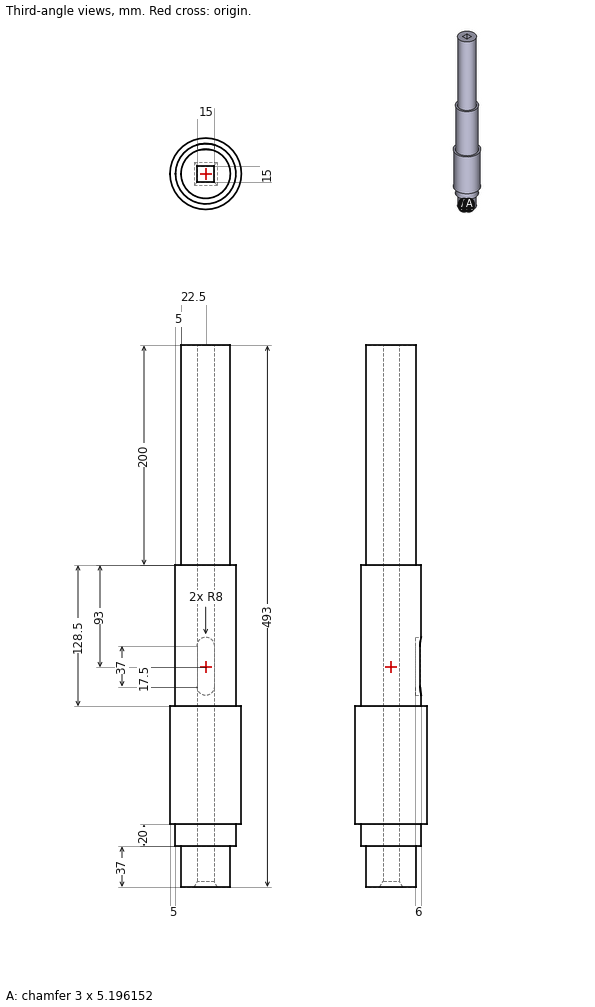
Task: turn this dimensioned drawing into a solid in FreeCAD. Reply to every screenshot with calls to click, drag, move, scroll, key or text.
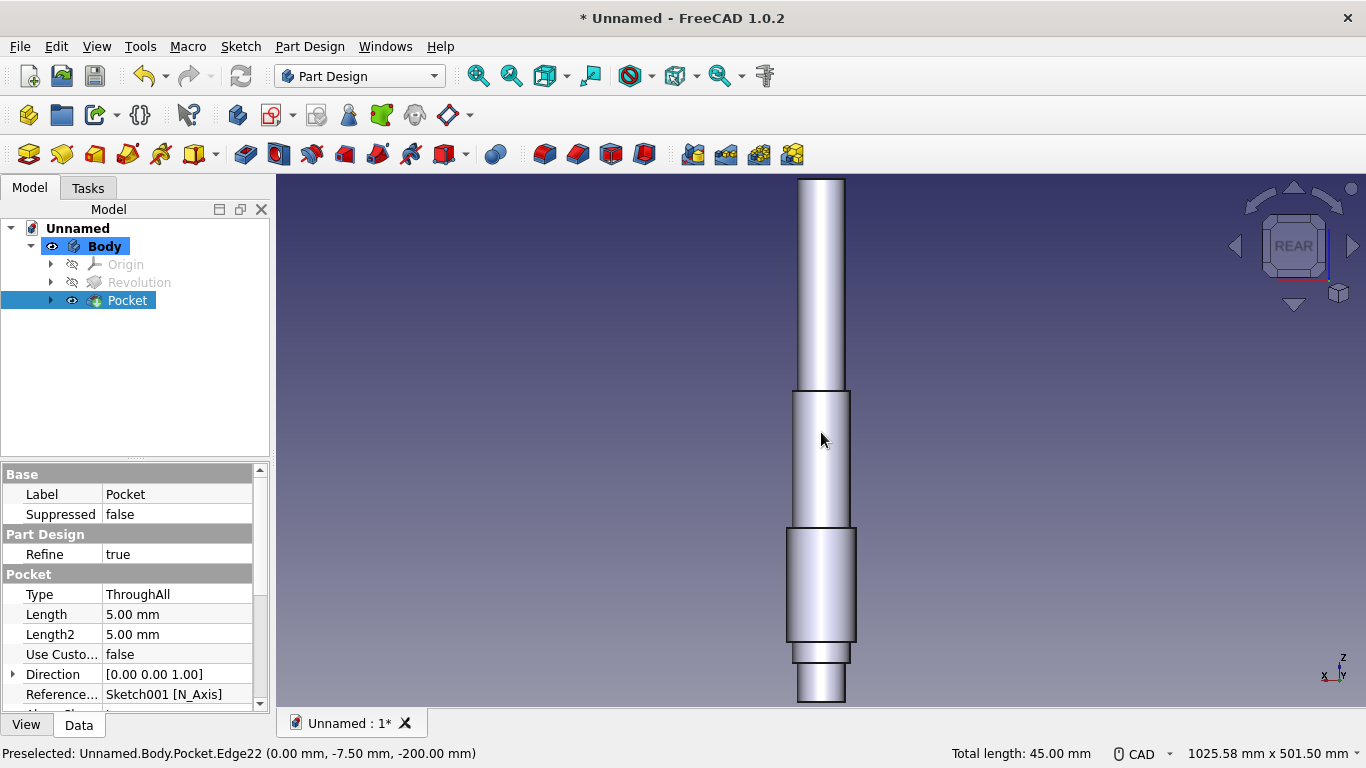
key(6)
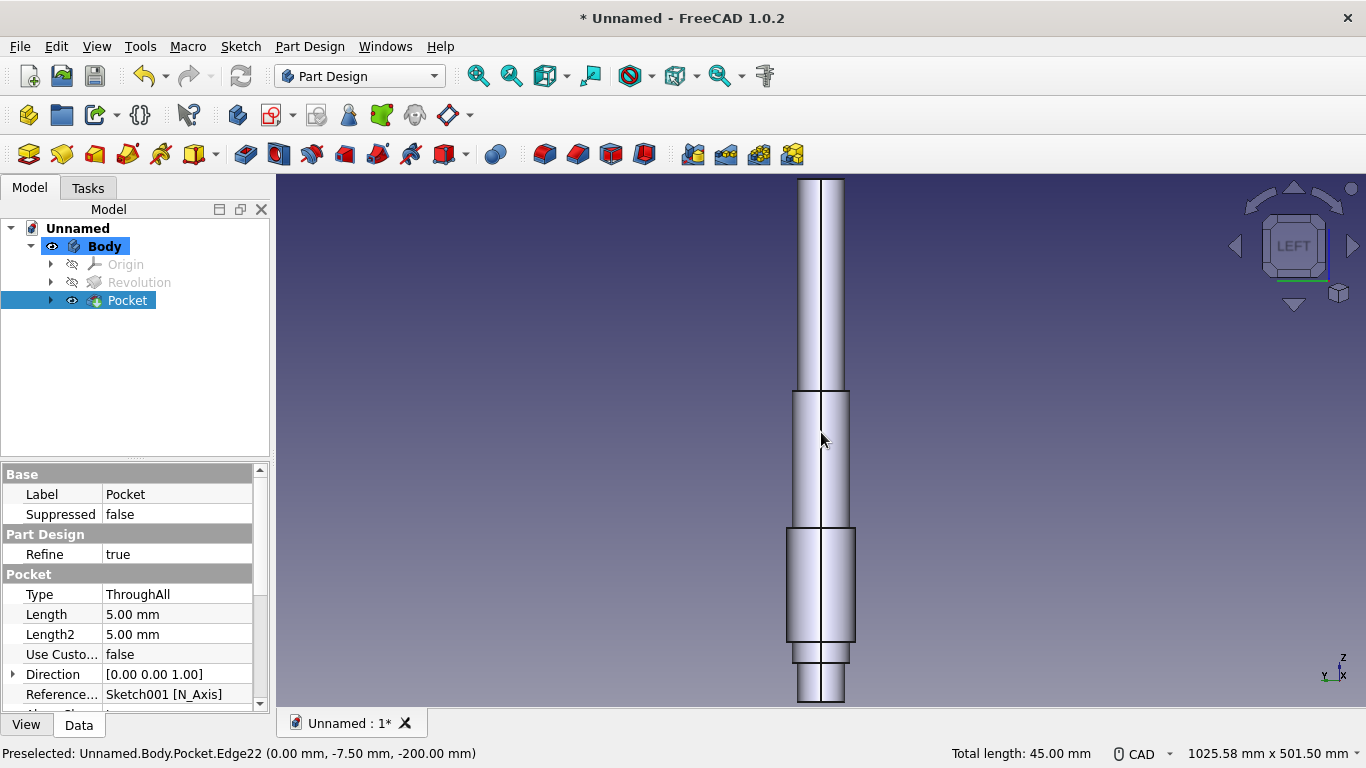
key(v)
key(3)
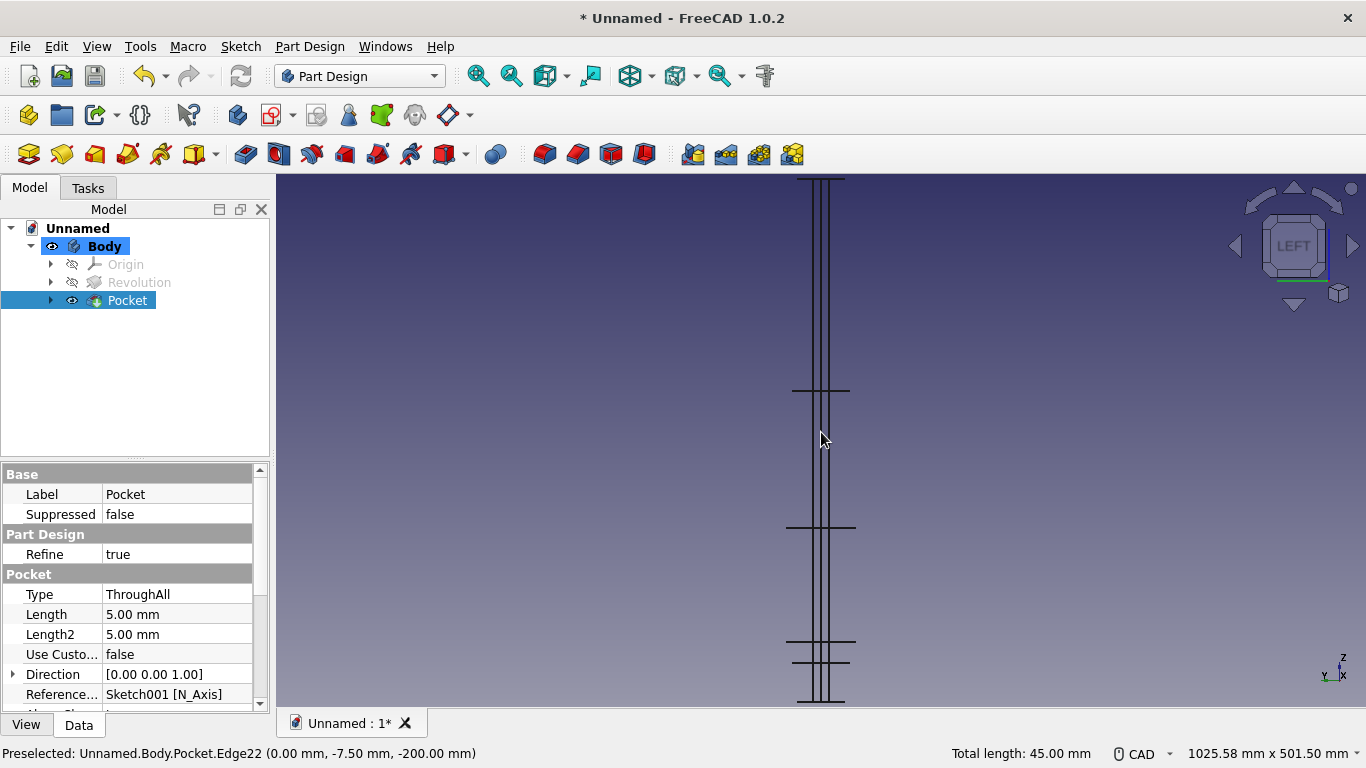
key(0)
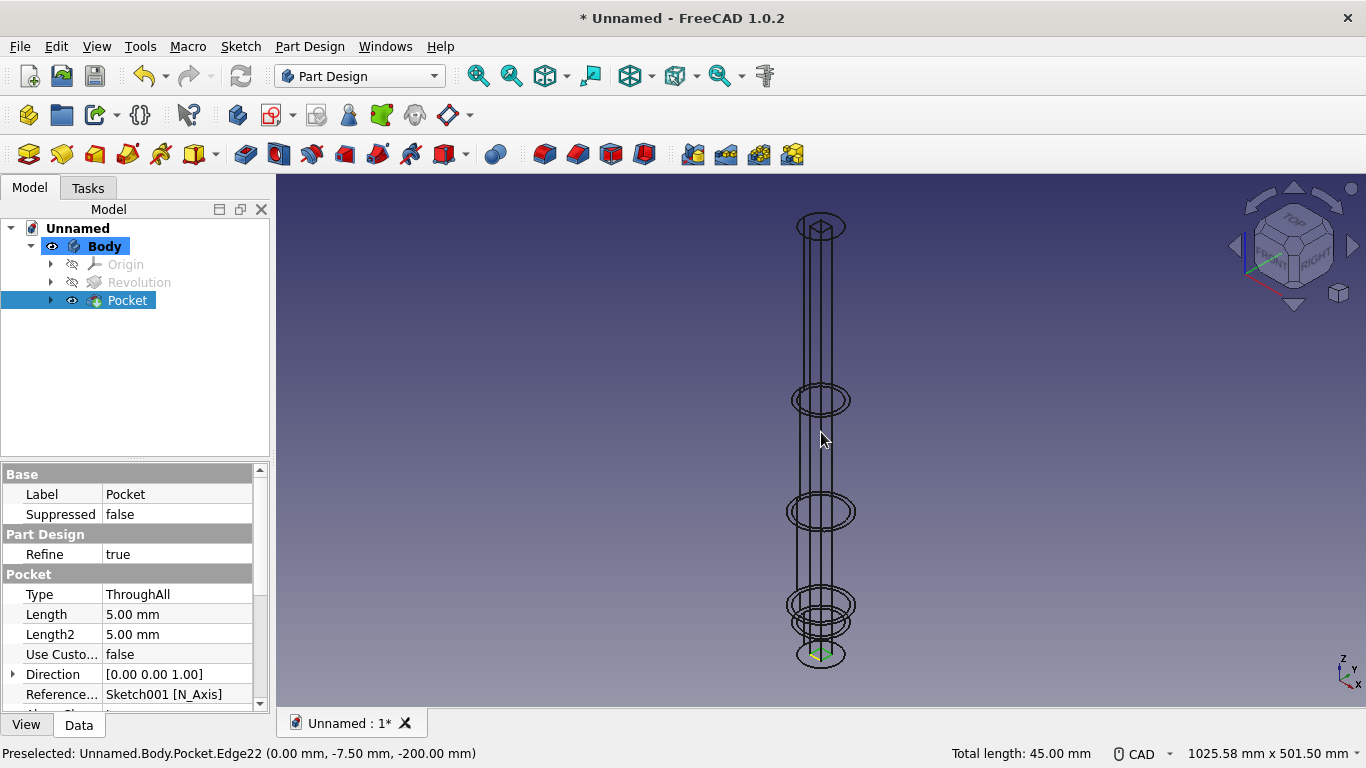
click(815, 657, ctrl)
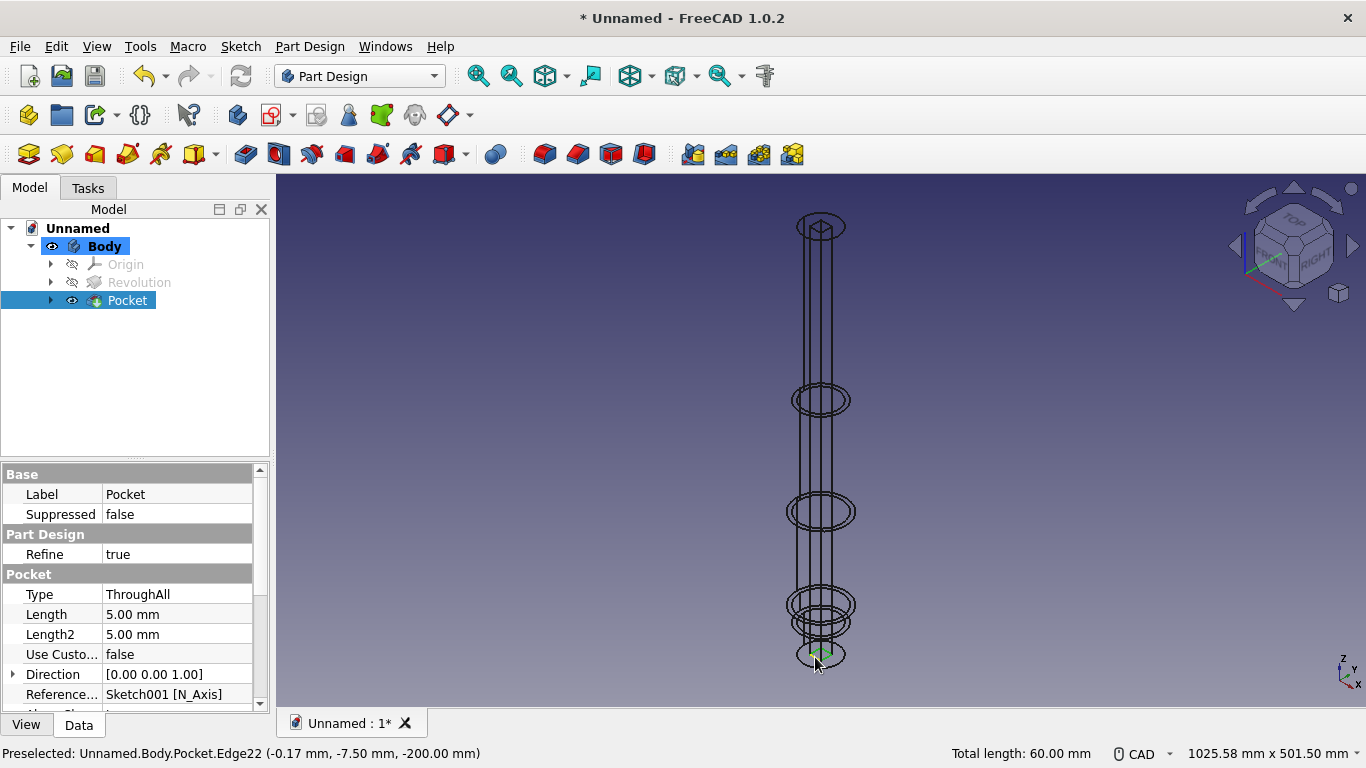
key(v)
key(1)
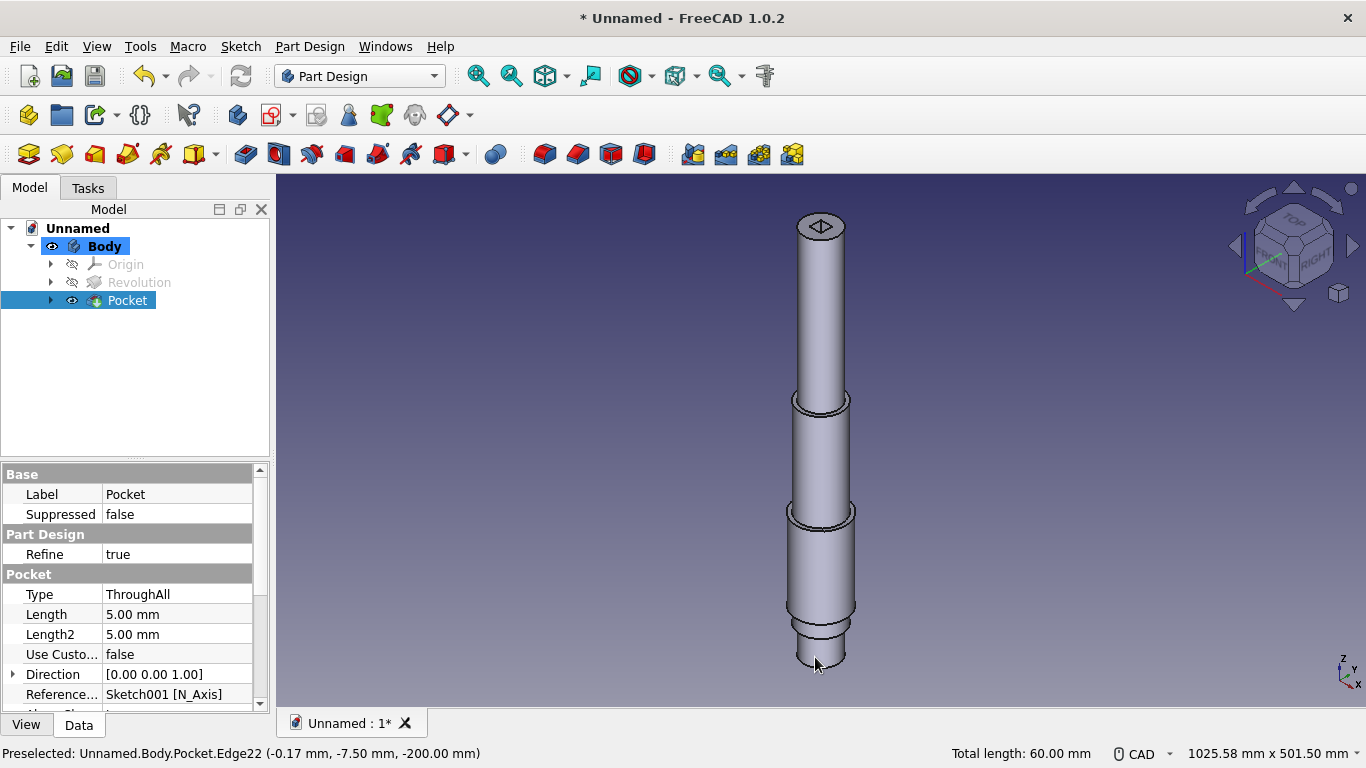
click(578, 154)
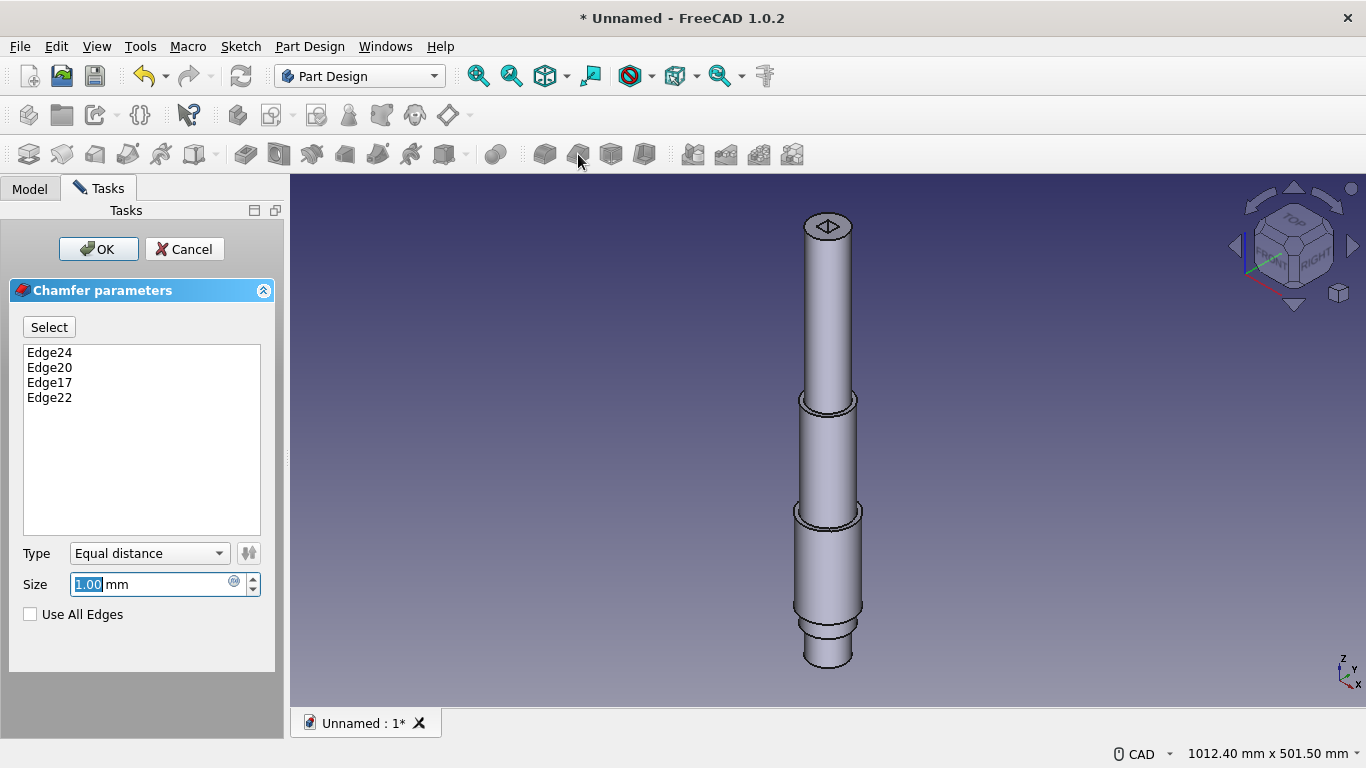
text(3)
key(Tab)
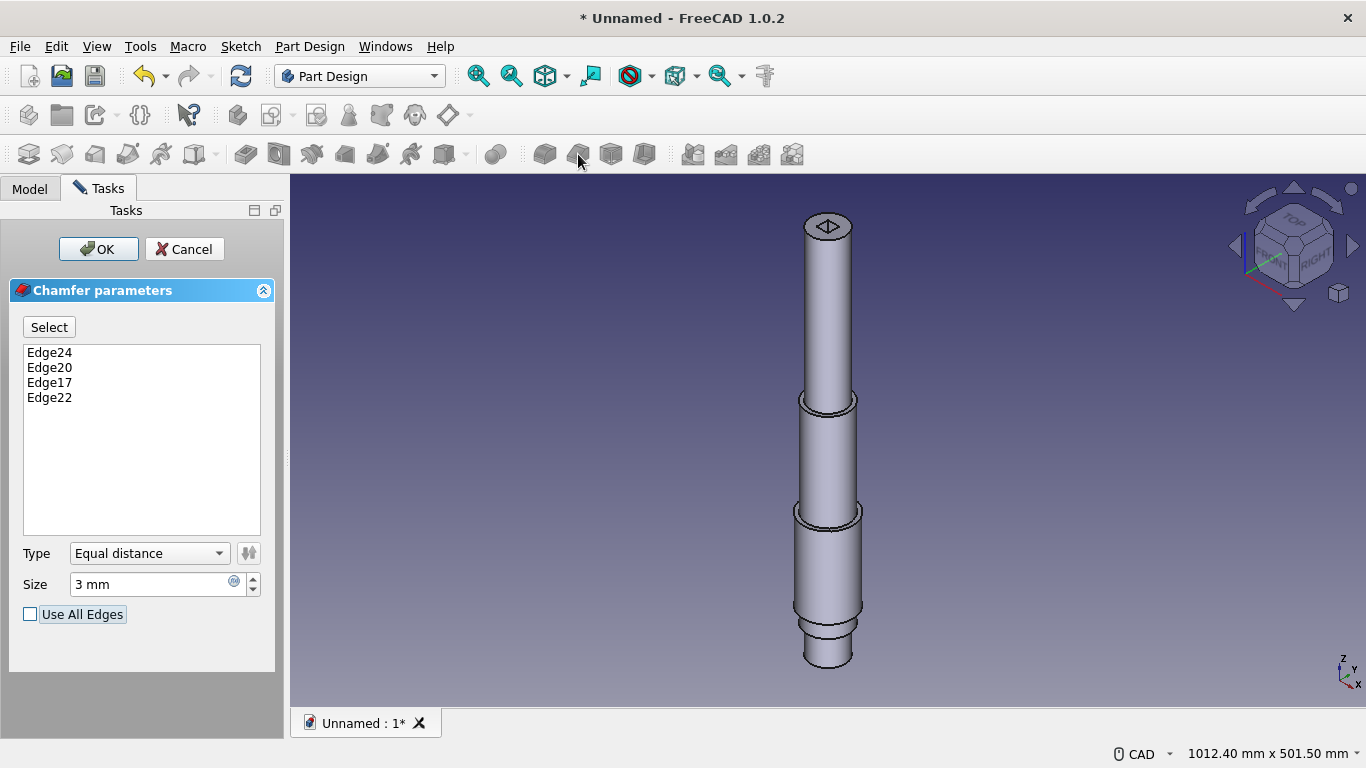
click(150, 554)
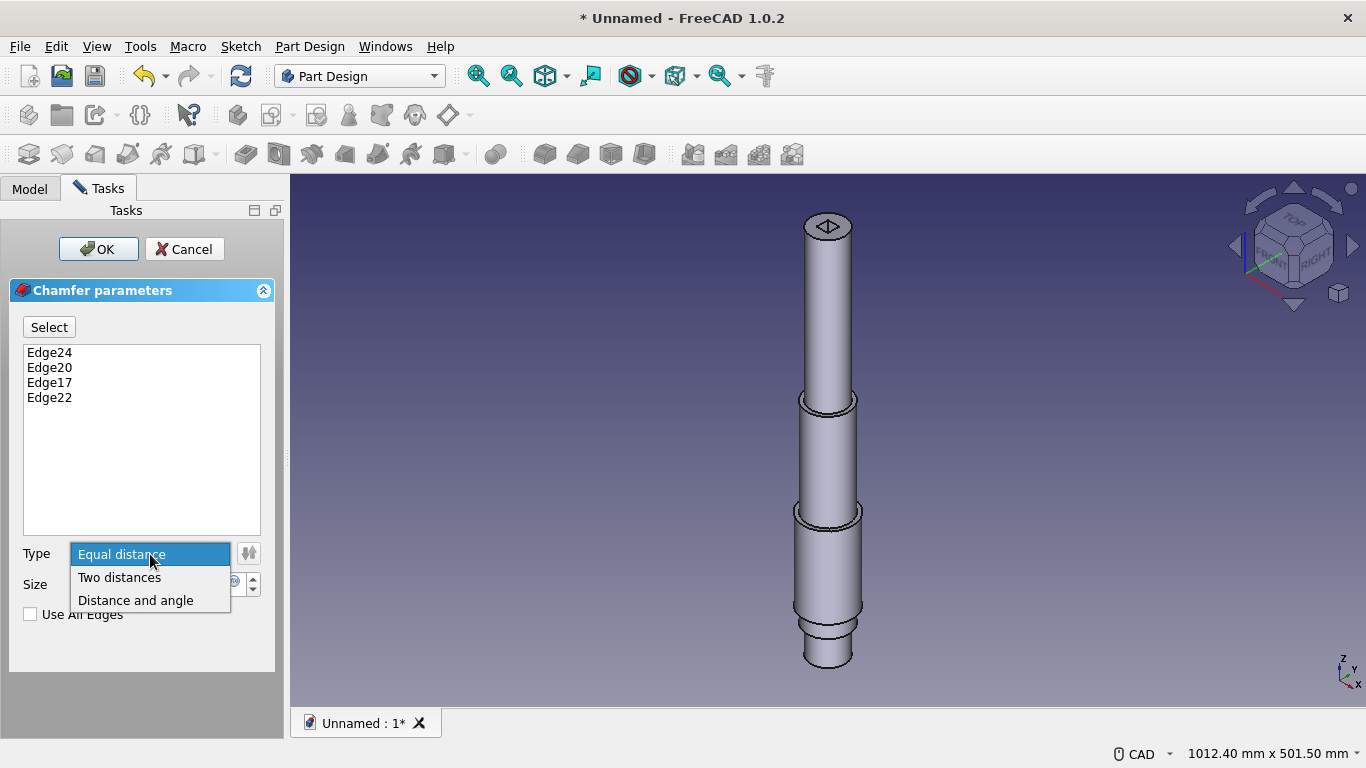
click(148, 578)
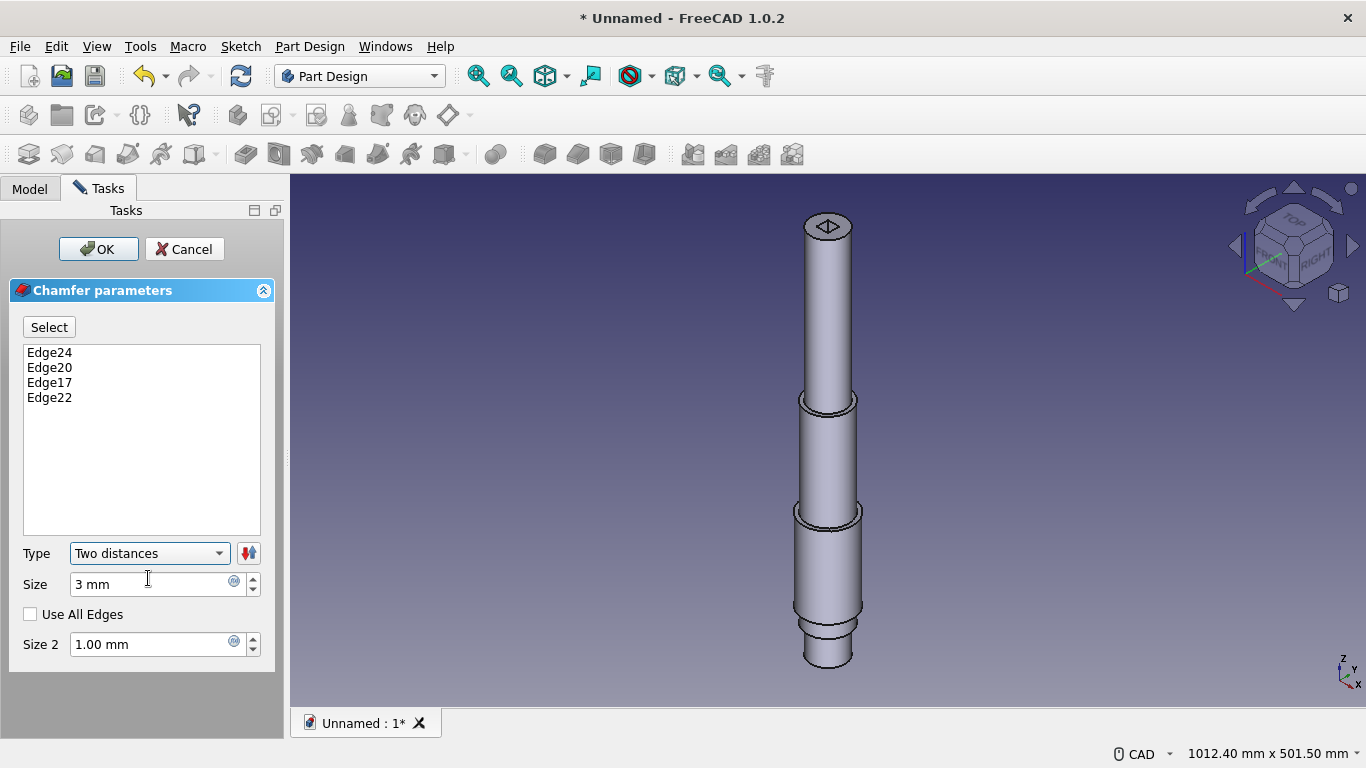
triple_click(158, 644)